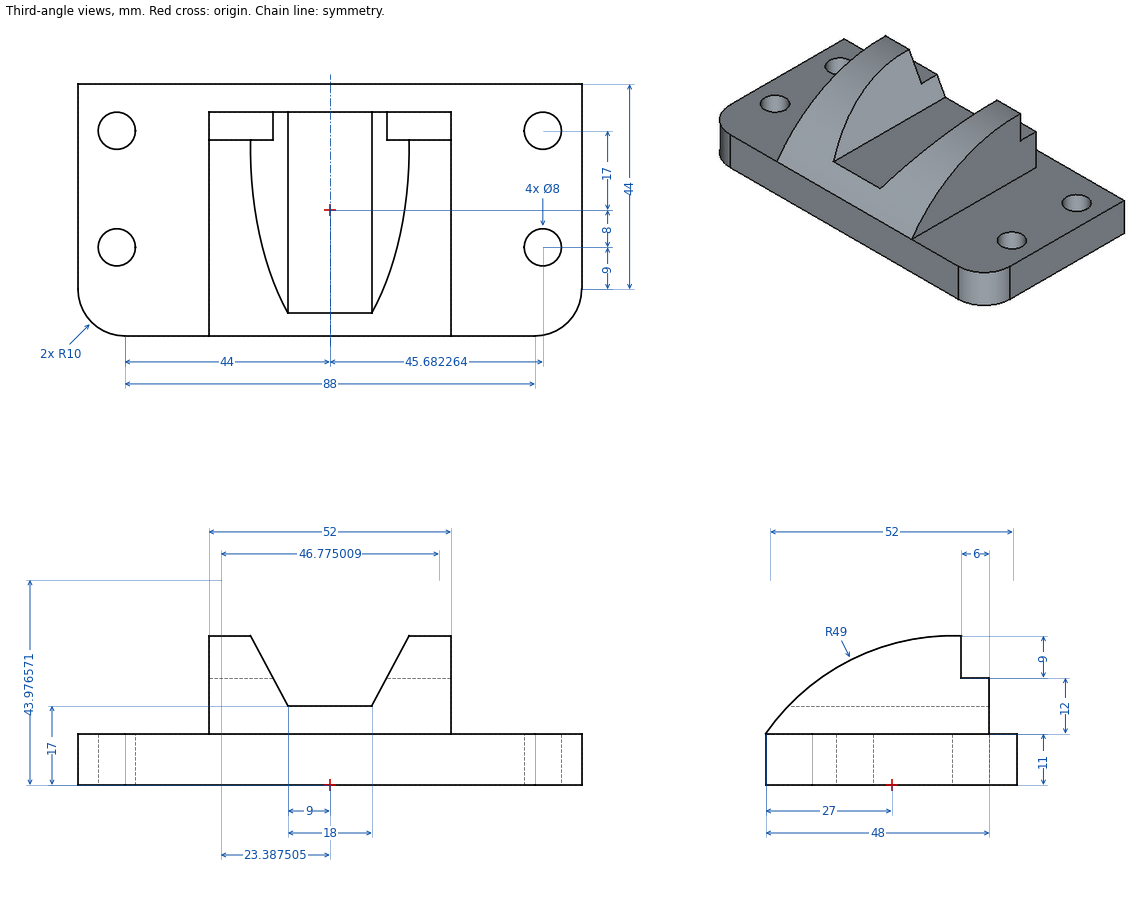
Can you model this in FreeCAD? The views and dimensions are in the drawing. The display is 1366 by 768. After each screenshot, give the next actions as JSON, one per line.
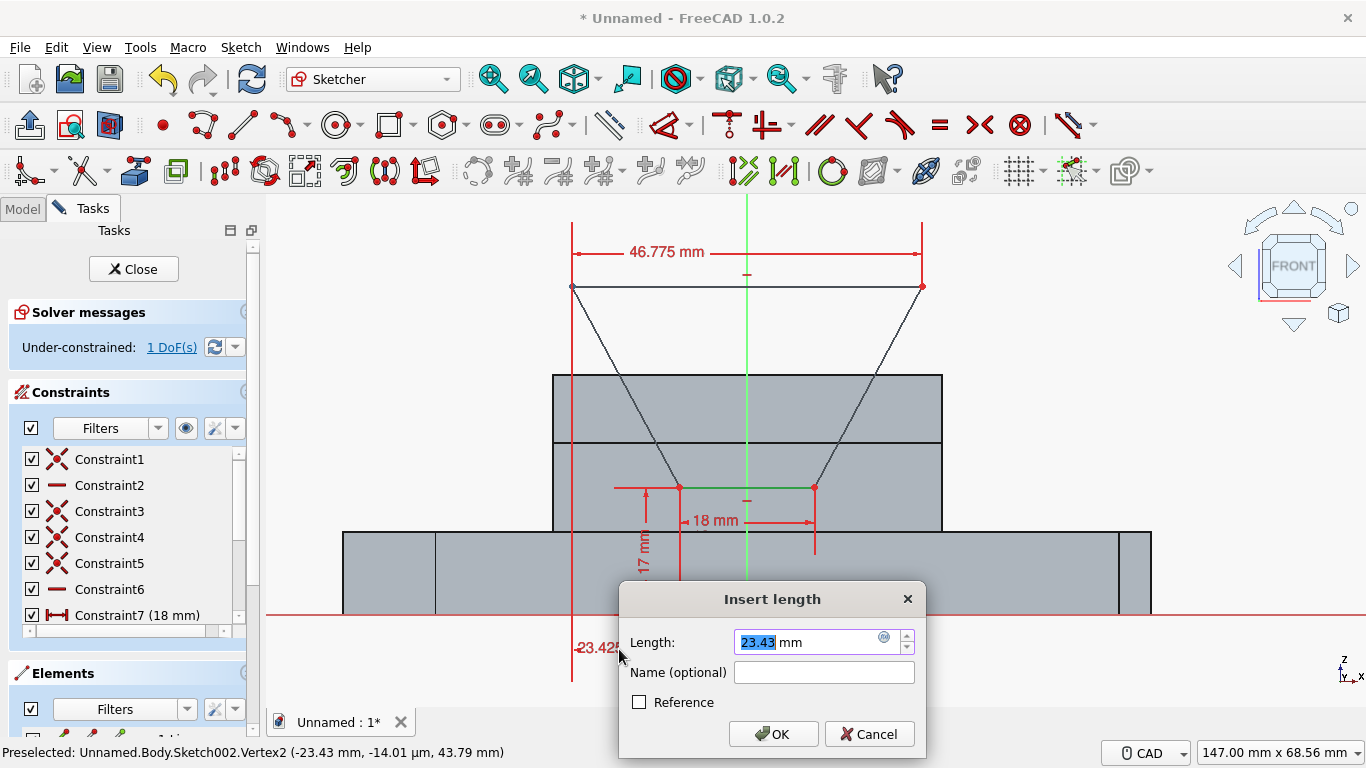
{"action": "type", "text": "23.387505"}
{"action": "key", "text": "Return"}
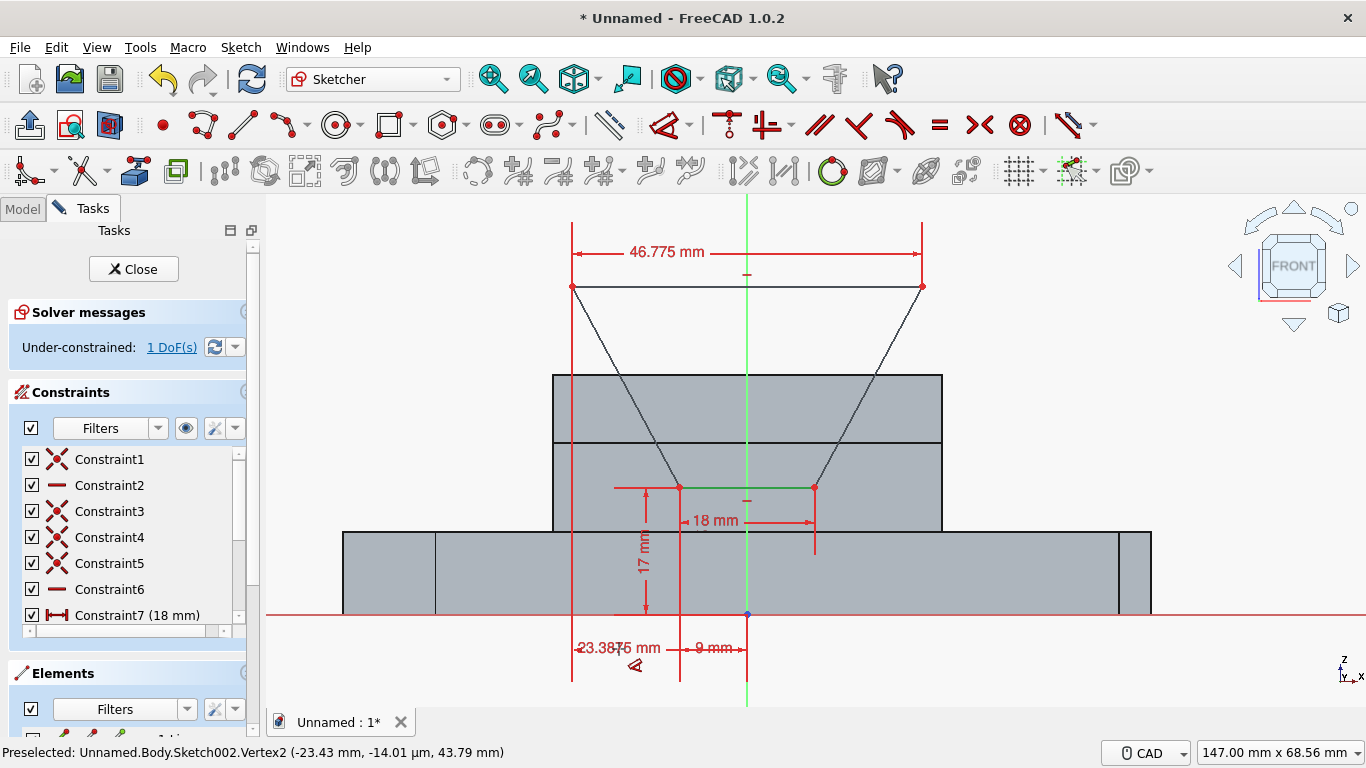
{"action": "left_click", "coordinate": [572, 287]}
{"action": "left_click", "coordinate": [538, 451]}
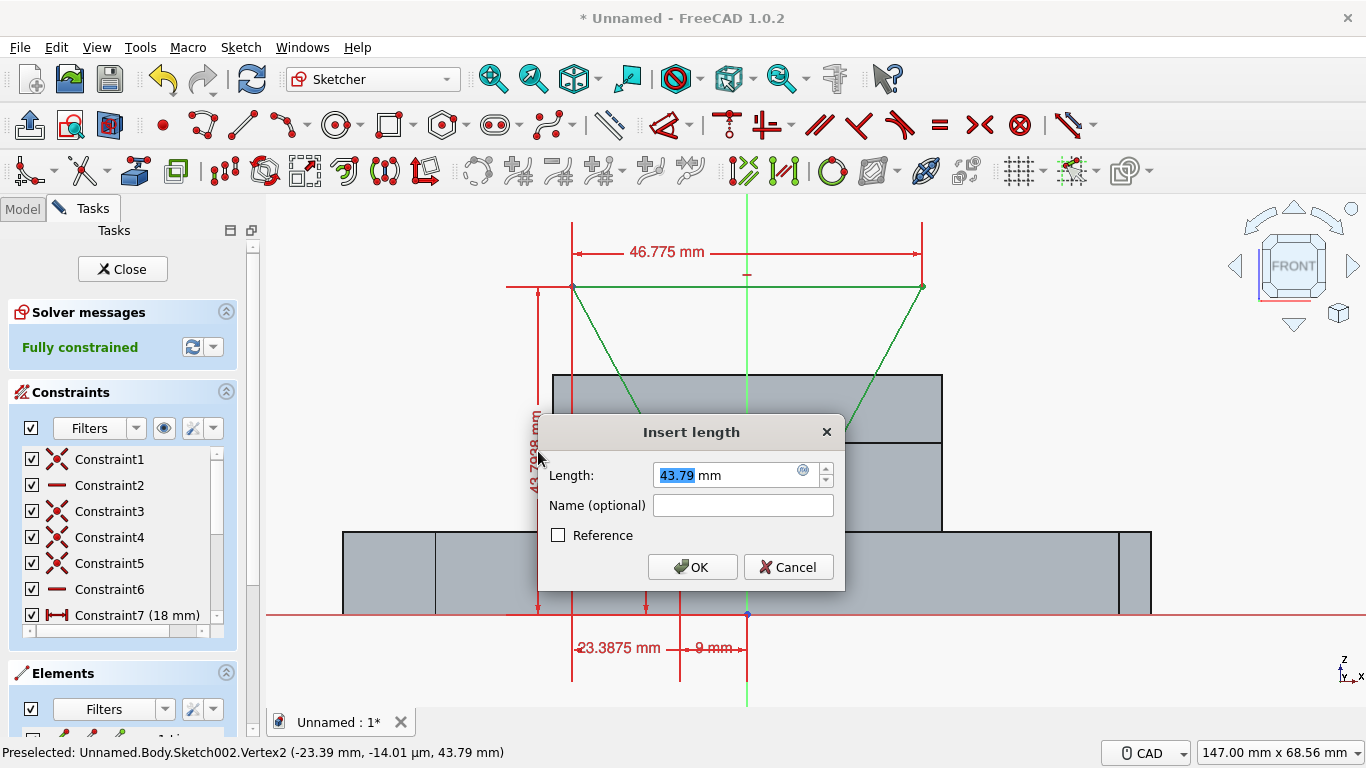
{"action": "type", "text": "43.976571"}
{"action": "key", "text": "Return"}
{"action": "key", "text": "Escape"}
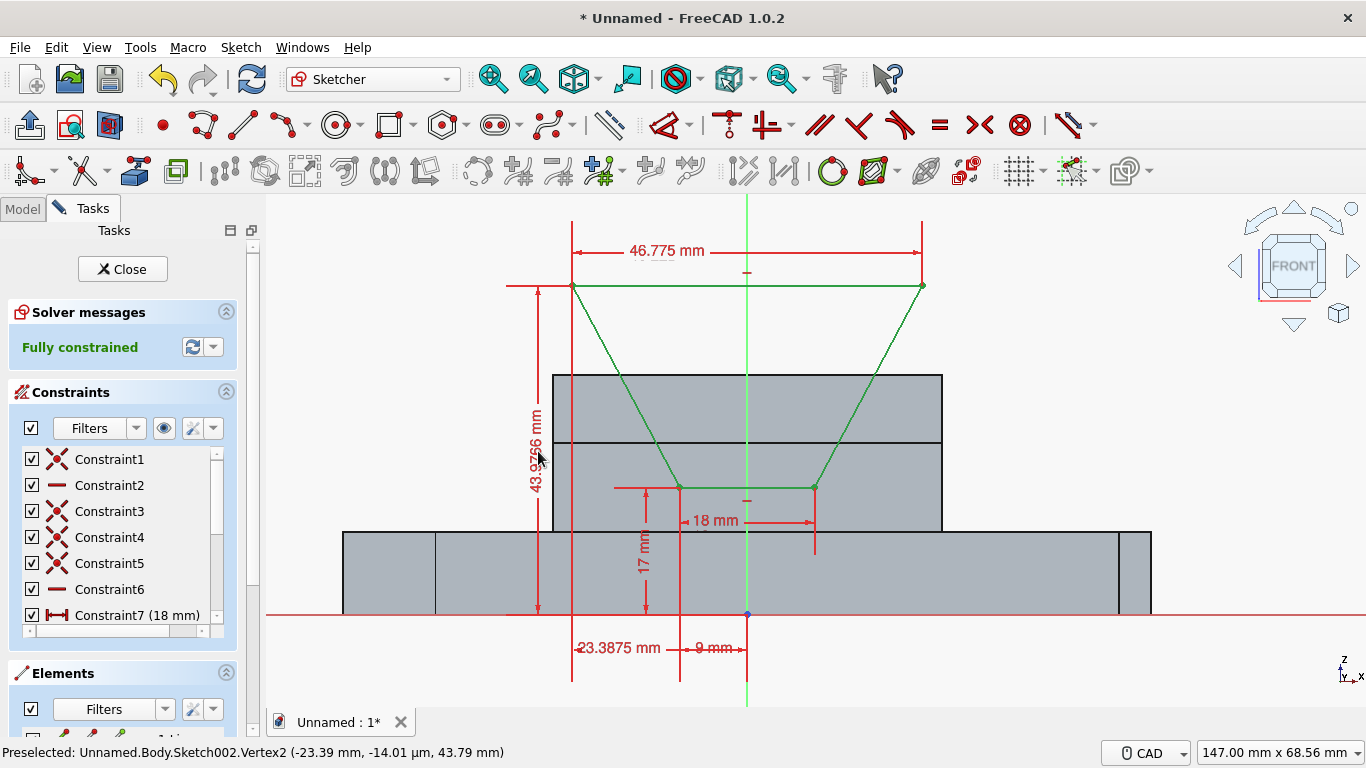
{"action": "left_click", "coordinate": [123, 269]}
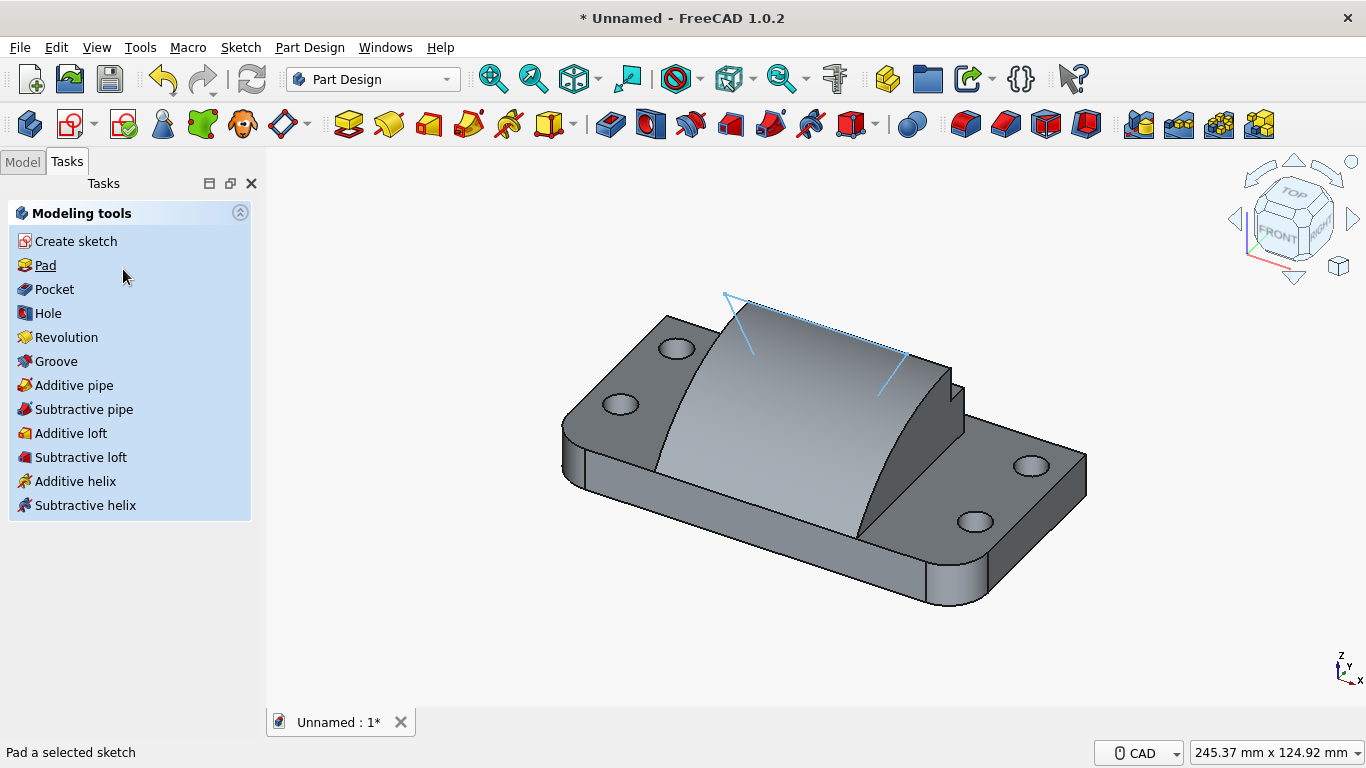
{"action": "left_click", "coordinate": [612, 124]}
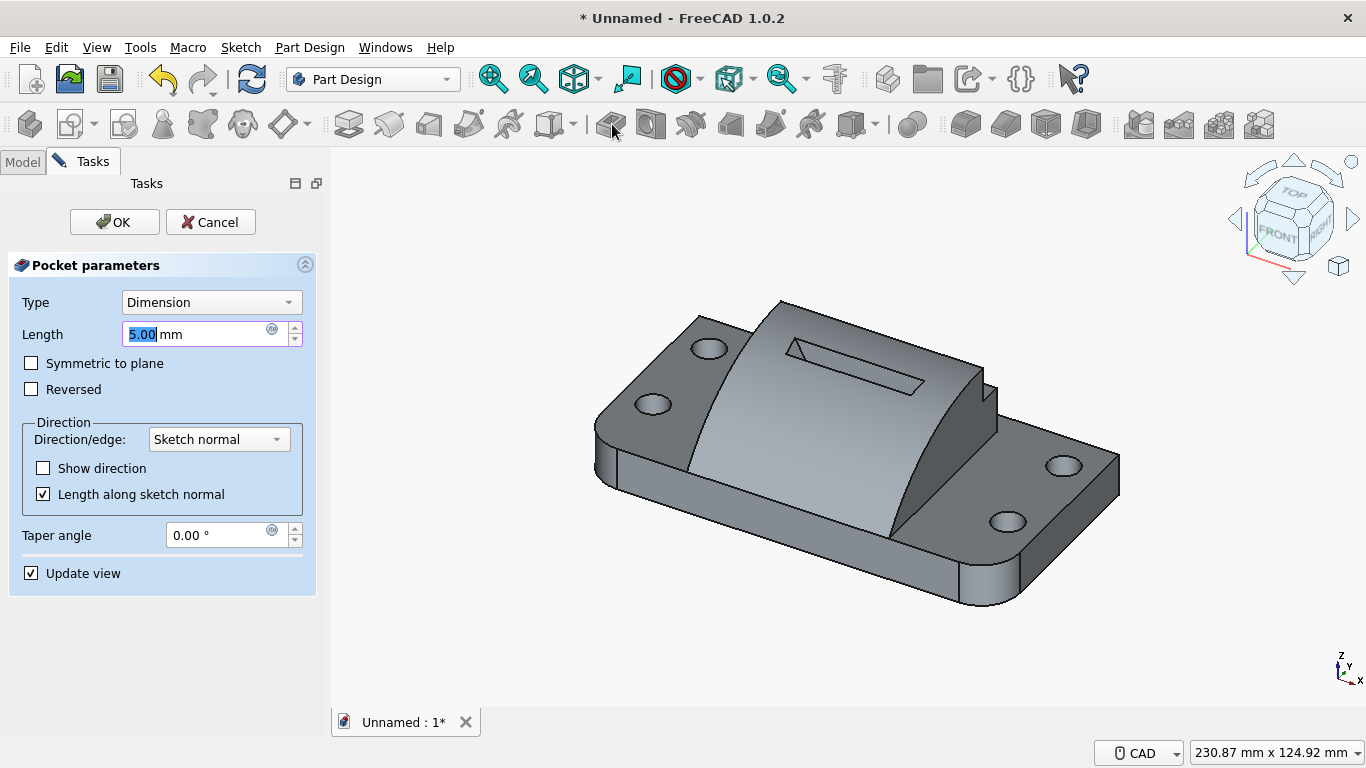
{"action": "type", "text": "52"}
{"action": "key", "text": "Tab"}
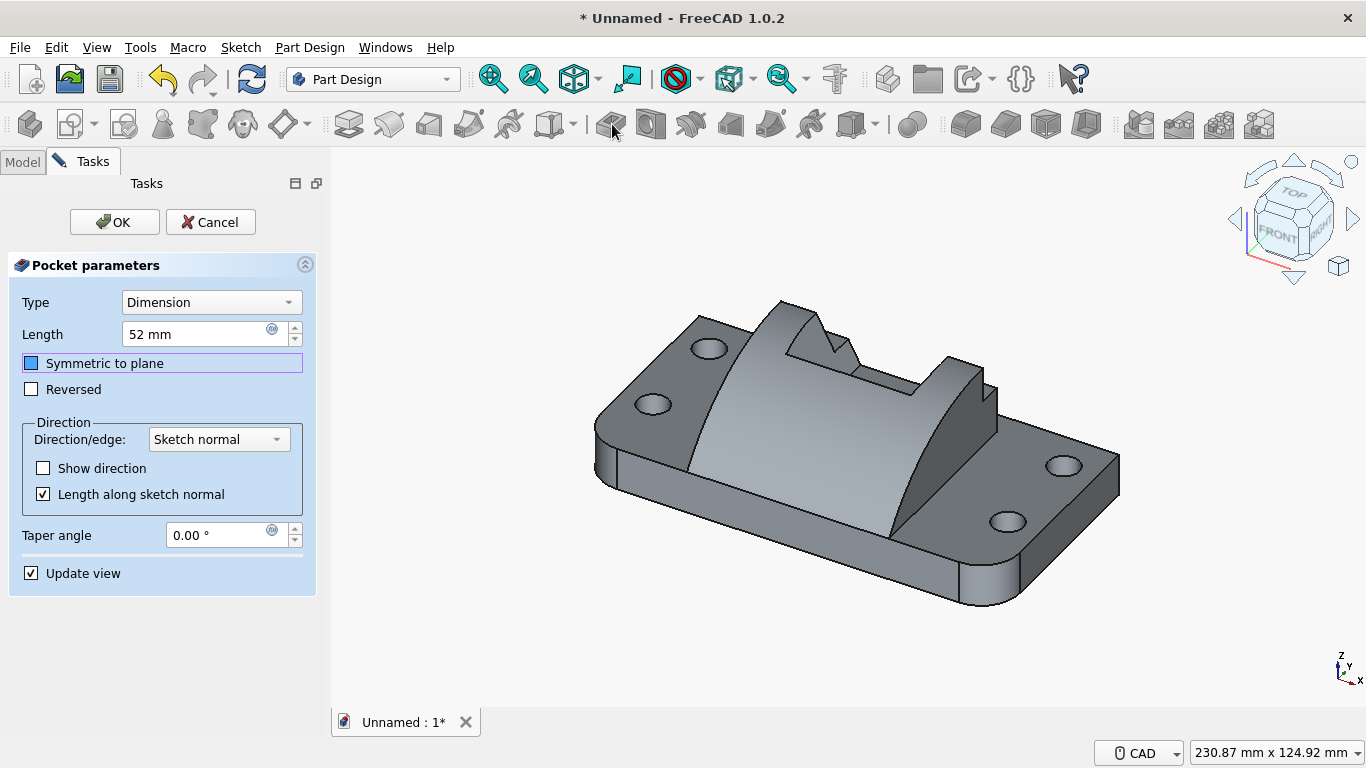
{"action": "left_click", "coordinate": [30, 363]}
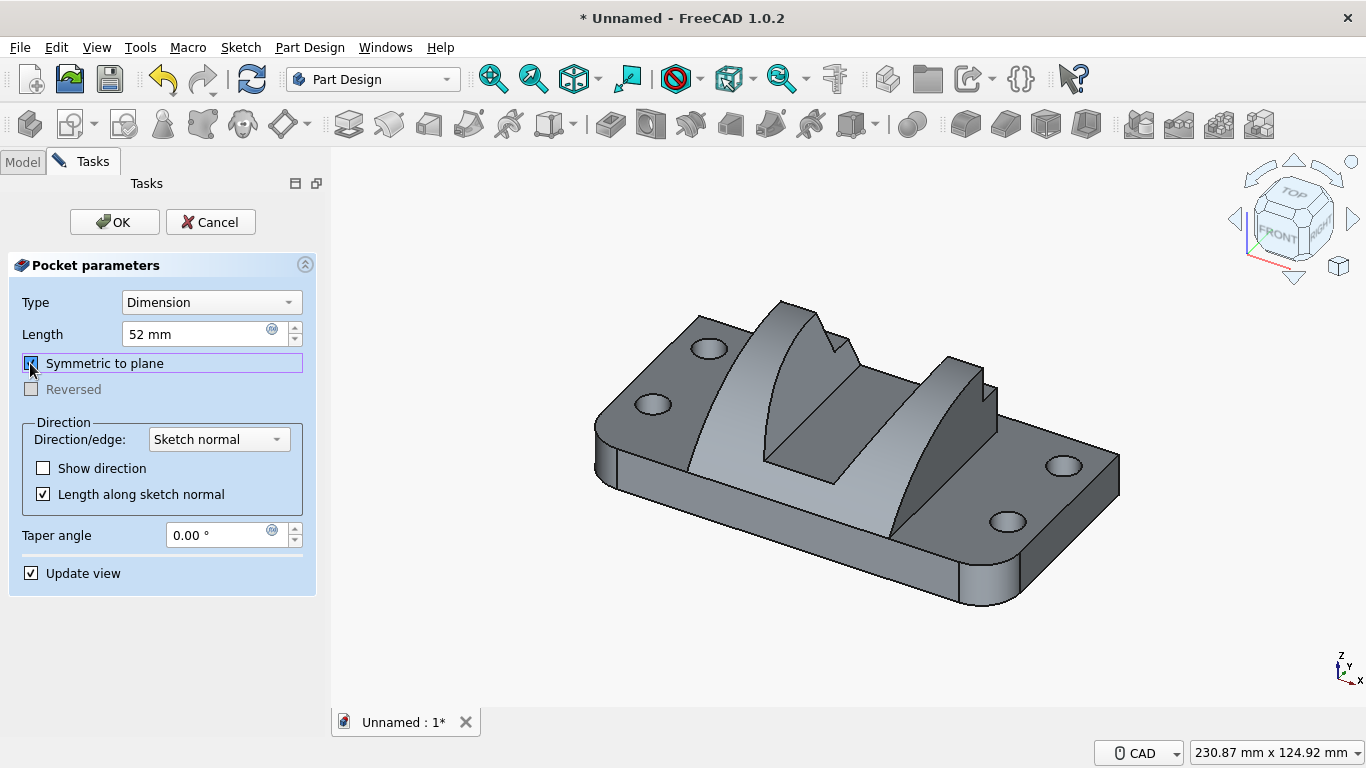
{"action": "left_click", "coordinate": [115, 222]}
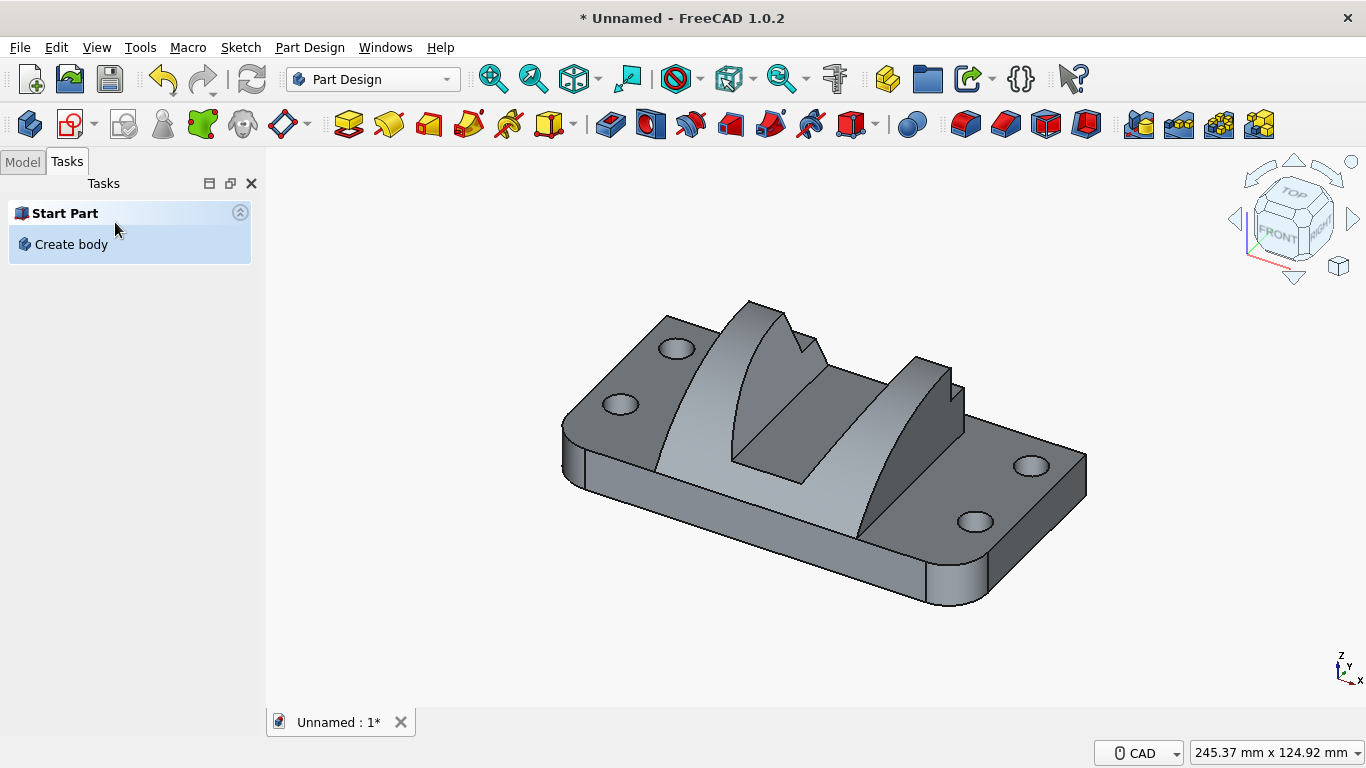
{"action": "key", "text": "0"}